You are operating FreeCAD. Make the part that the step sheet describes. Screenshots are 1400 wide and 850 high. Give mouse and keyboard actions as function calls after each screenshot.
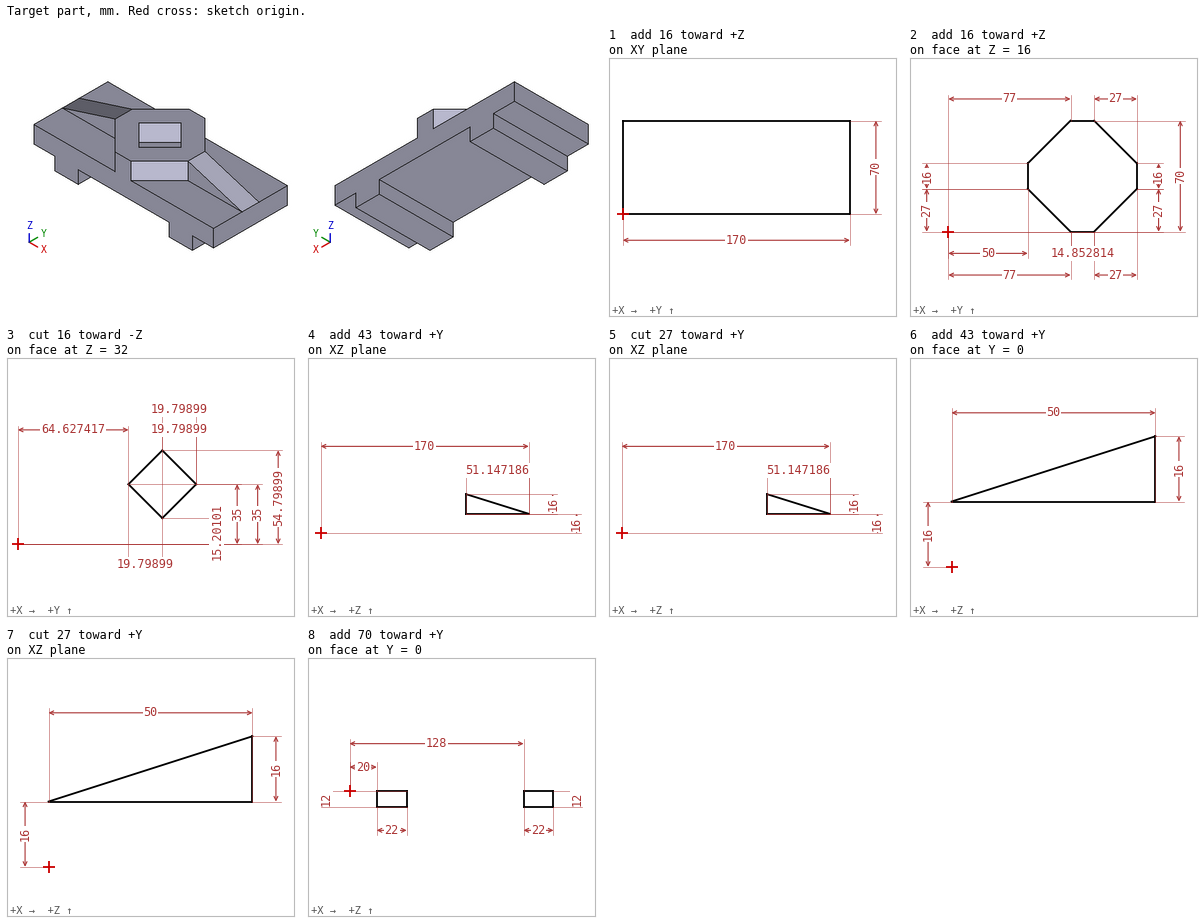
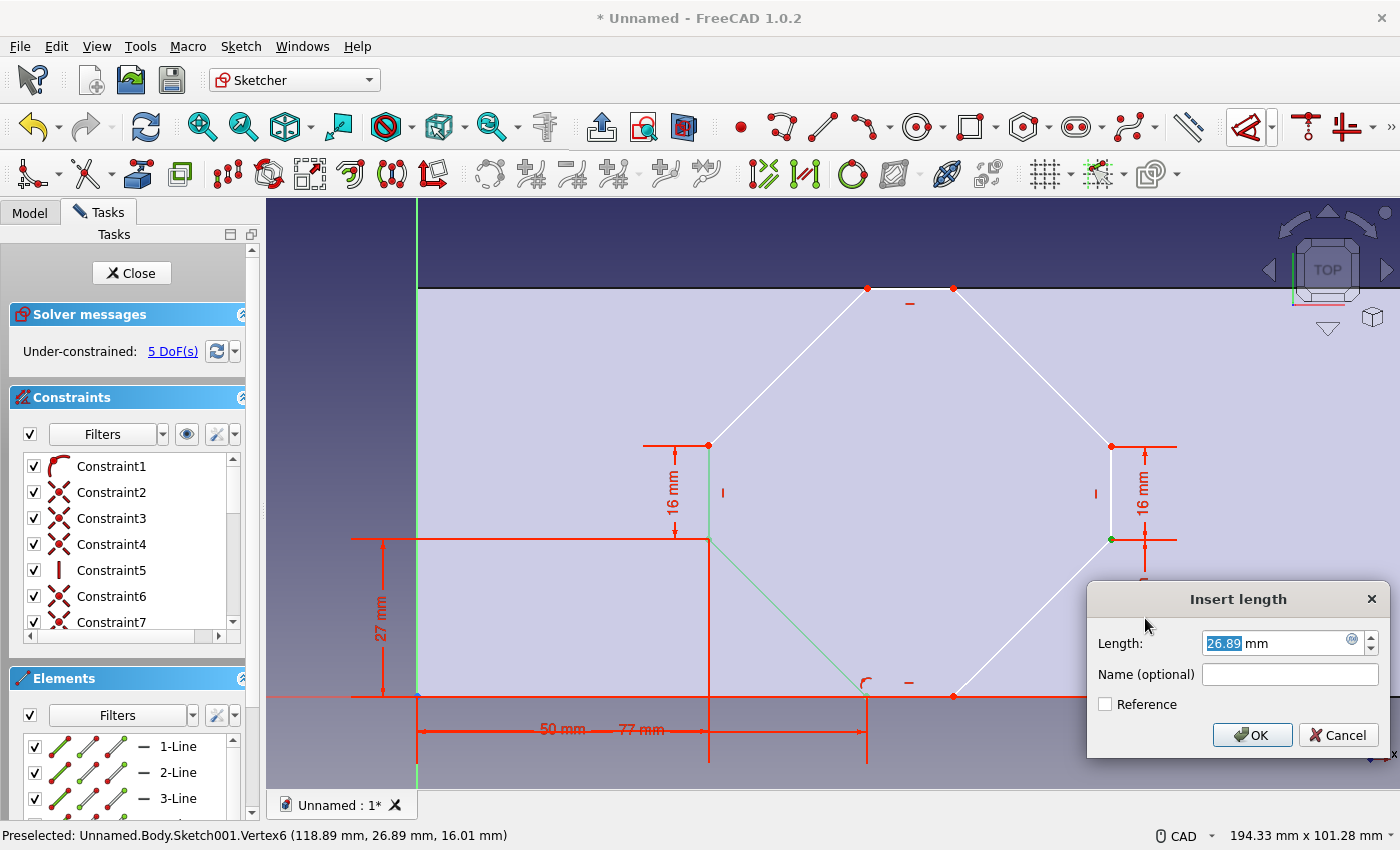
text(27)
key(Return)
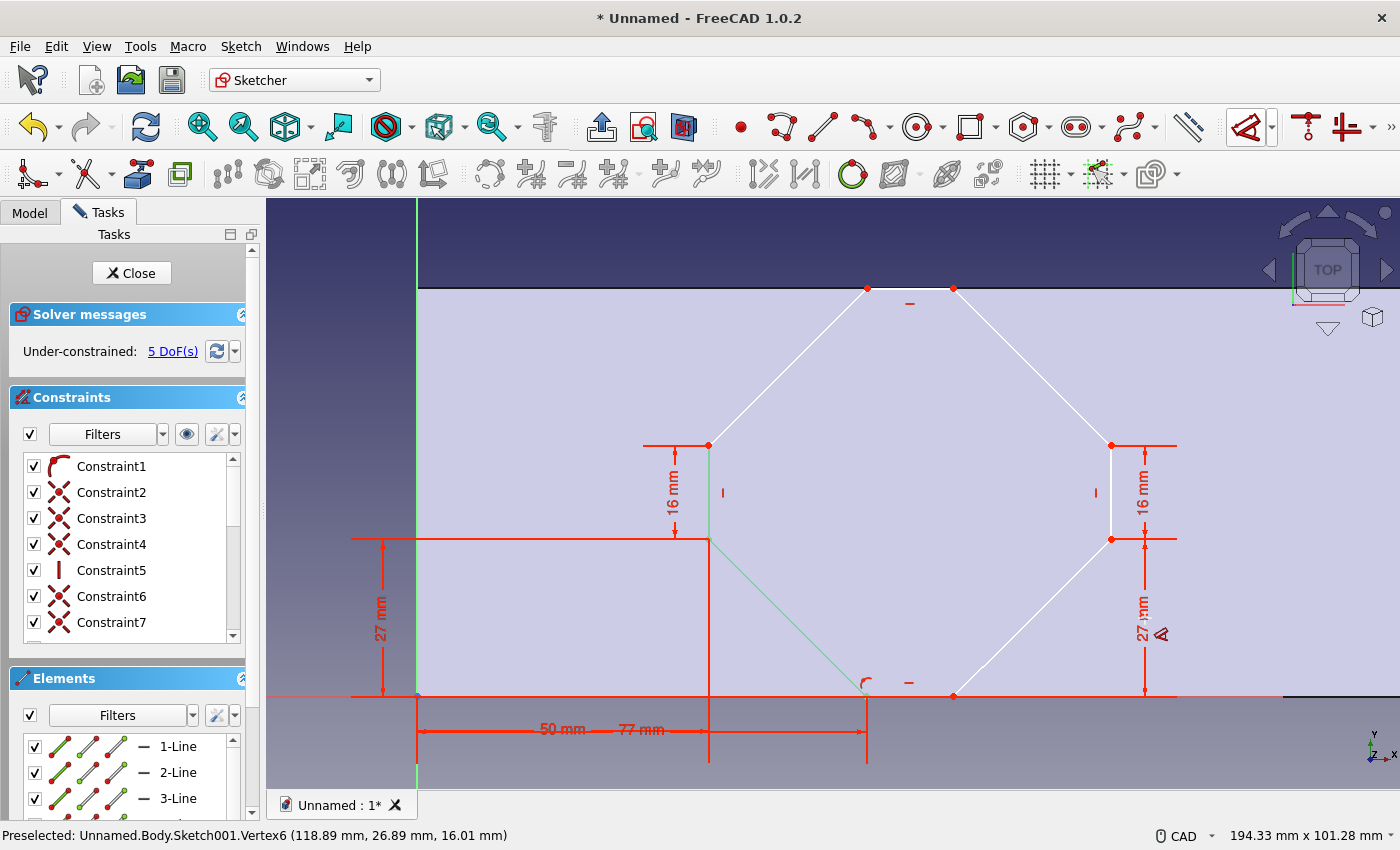
click(953, 289)
click(383, 493)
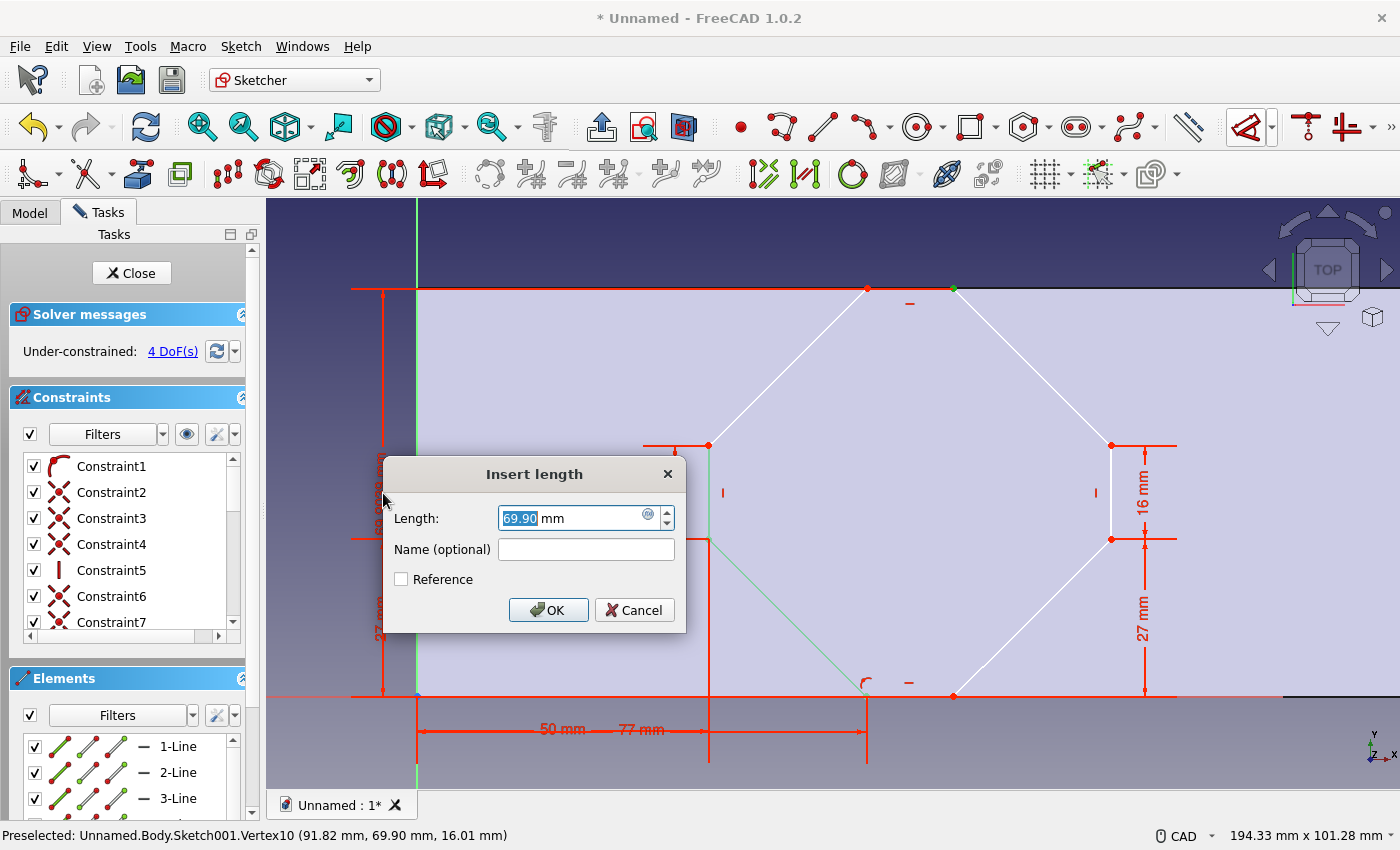
text(70)
key(Return)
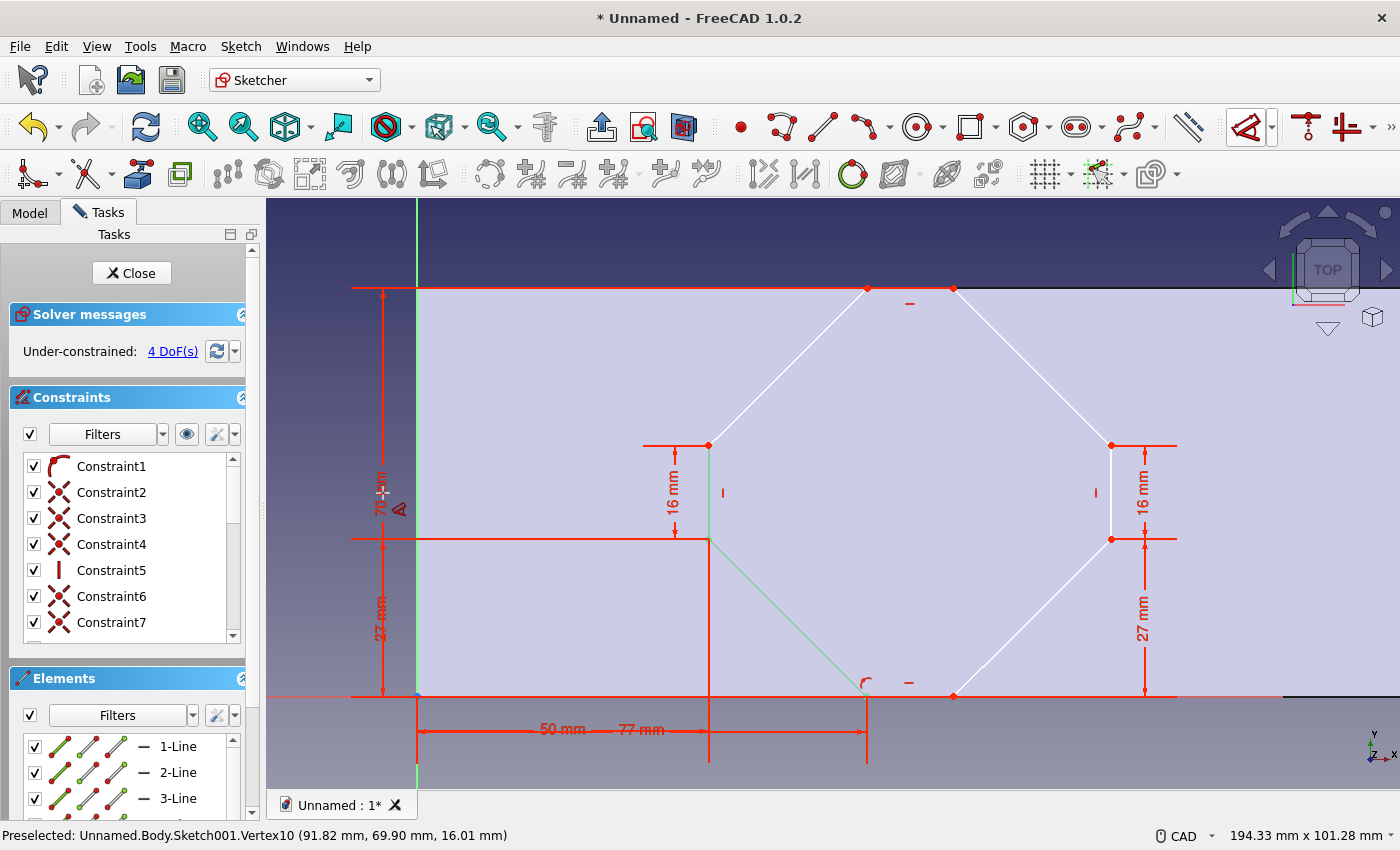
click(867, 288)
click(746, 731)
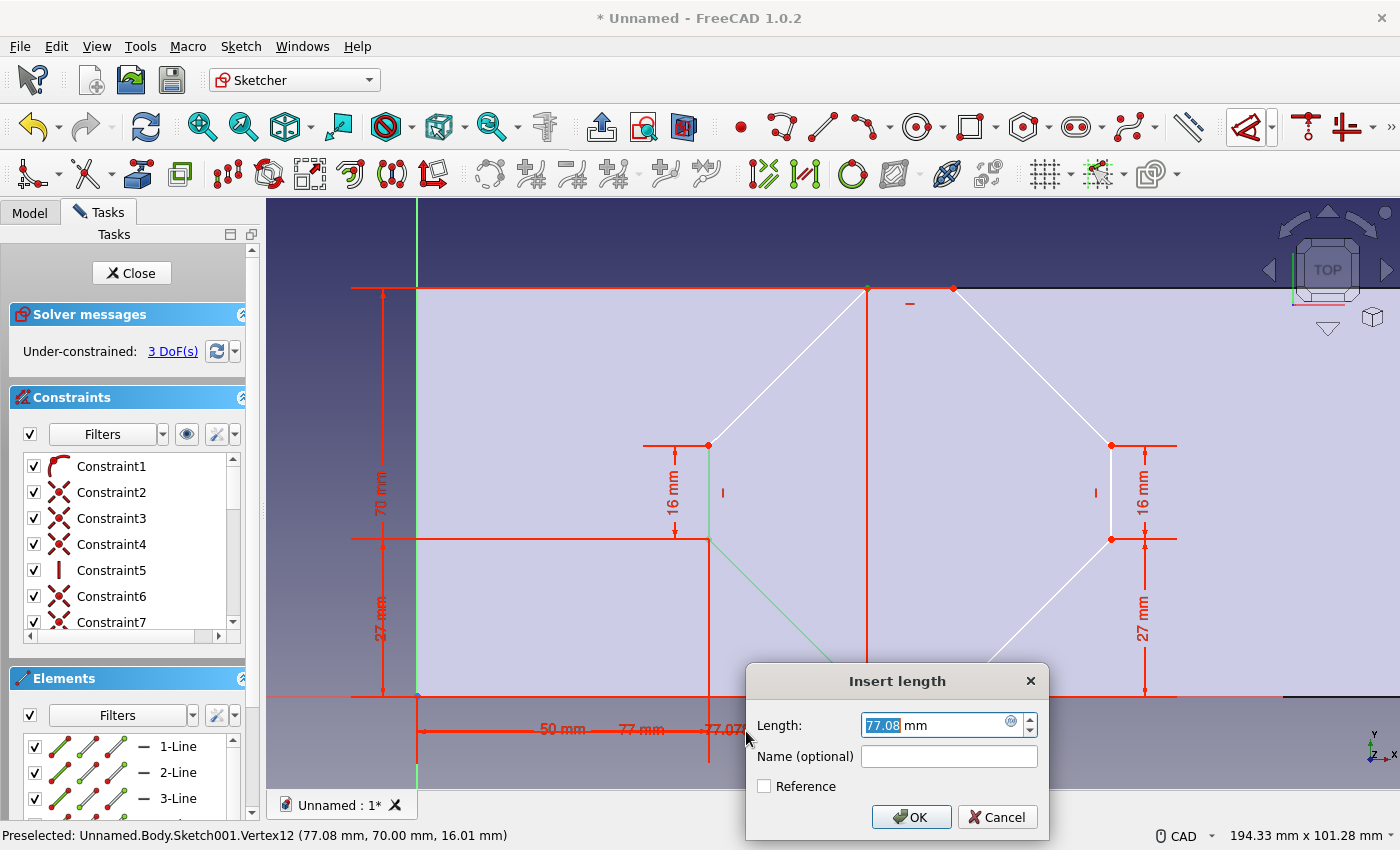
text(77)
key(Return)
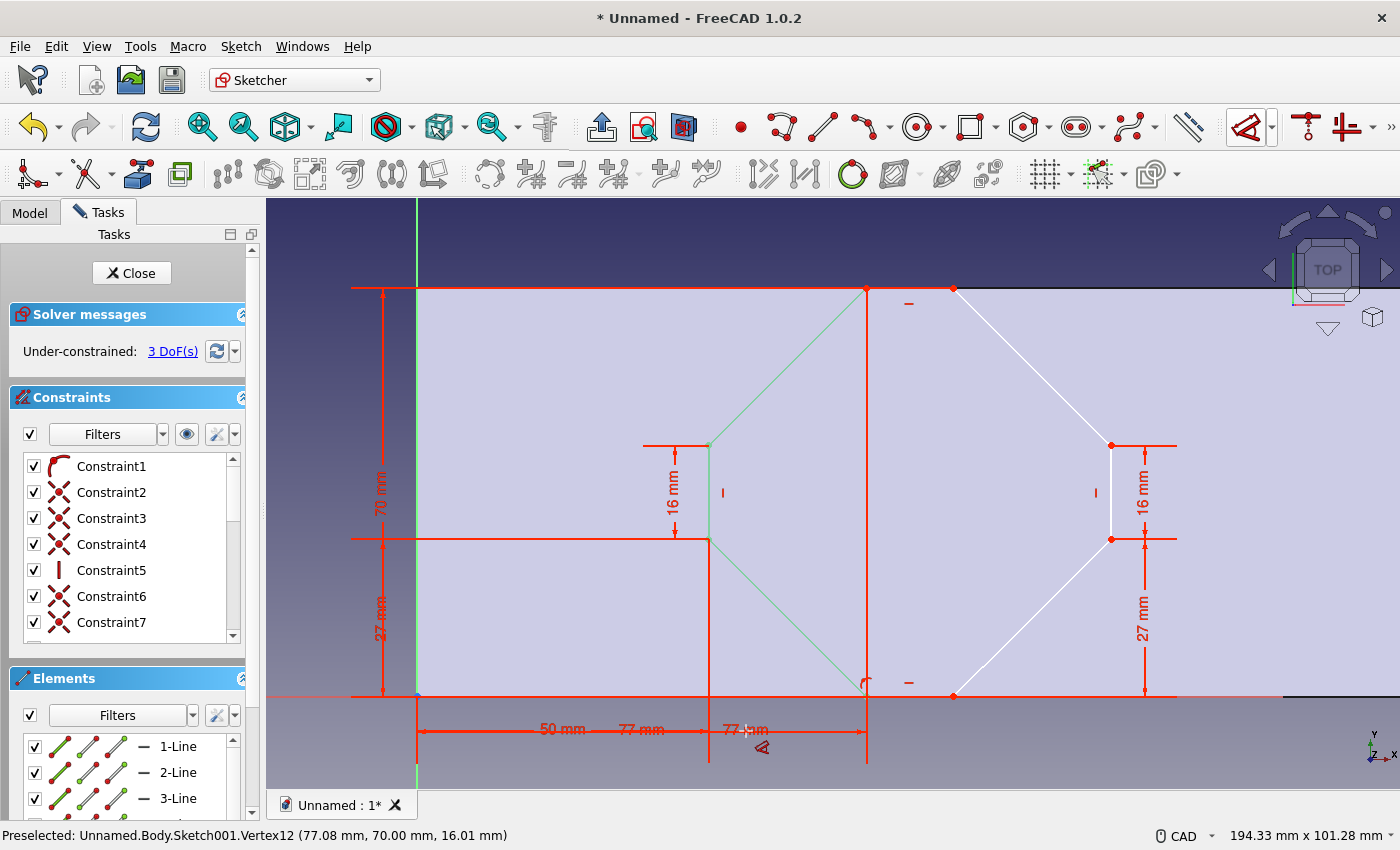
click(1000, 650)
click(1032, 731)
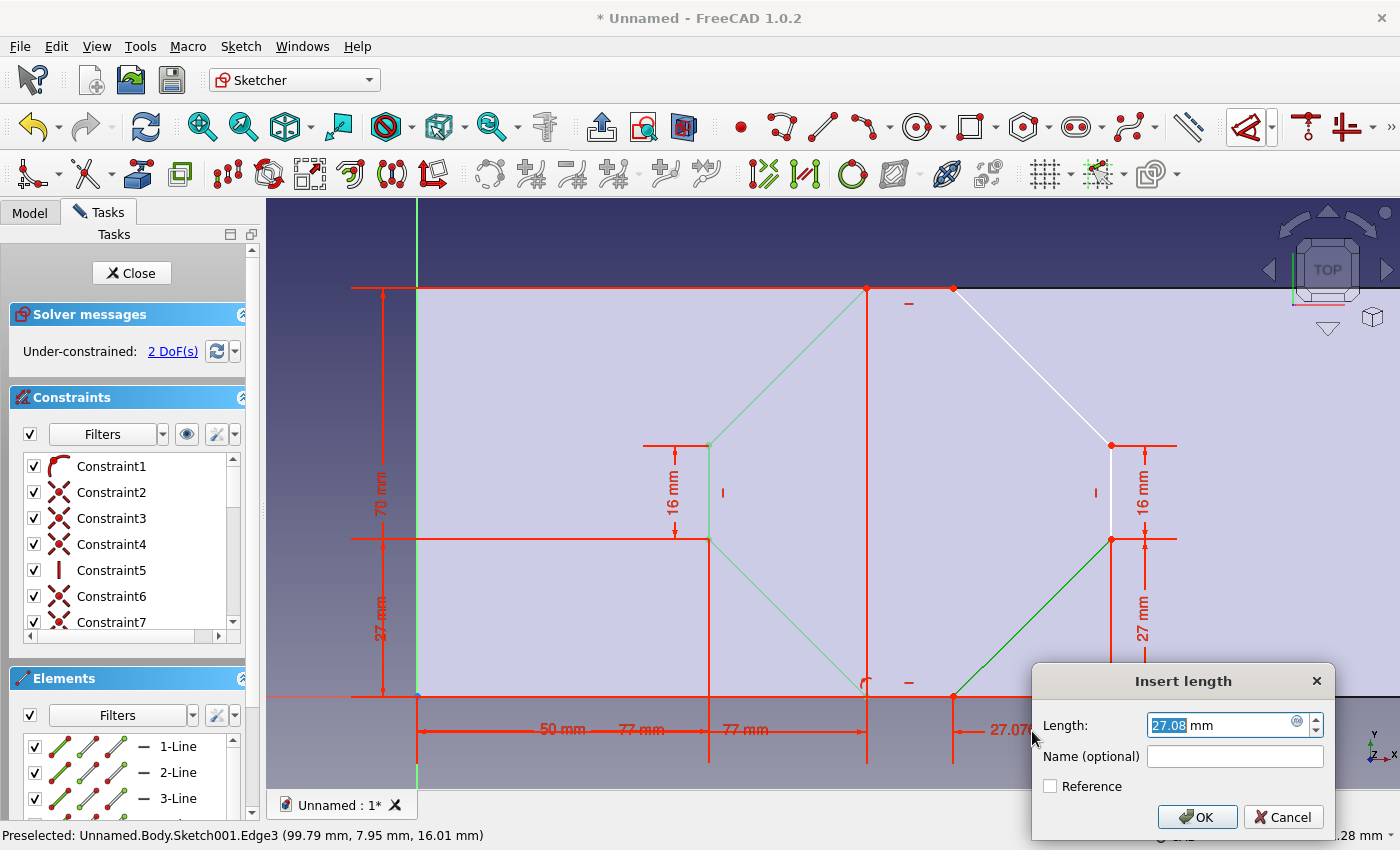
text(27)
key(Return)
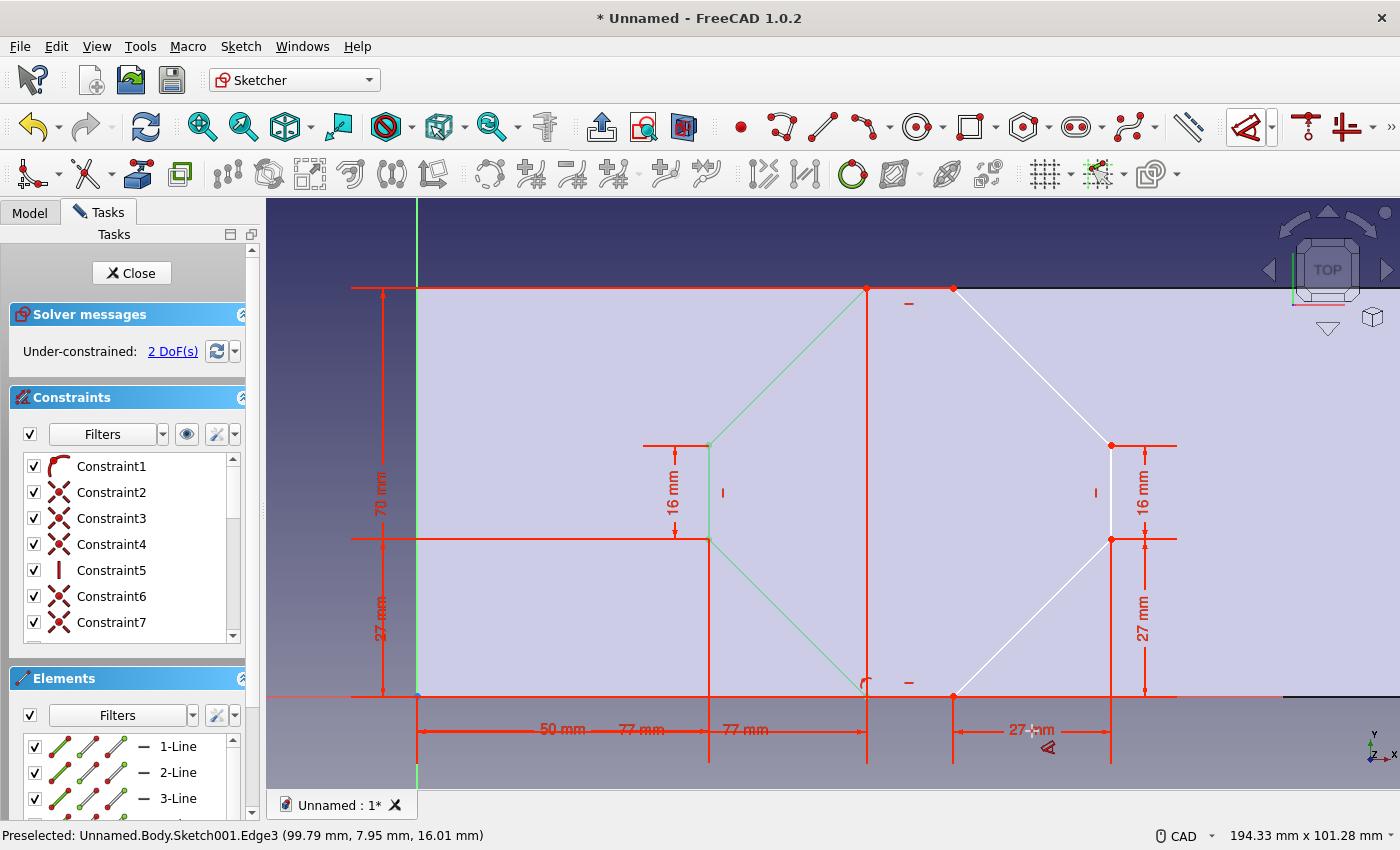
click(1064, 399)
click(1032, 254)